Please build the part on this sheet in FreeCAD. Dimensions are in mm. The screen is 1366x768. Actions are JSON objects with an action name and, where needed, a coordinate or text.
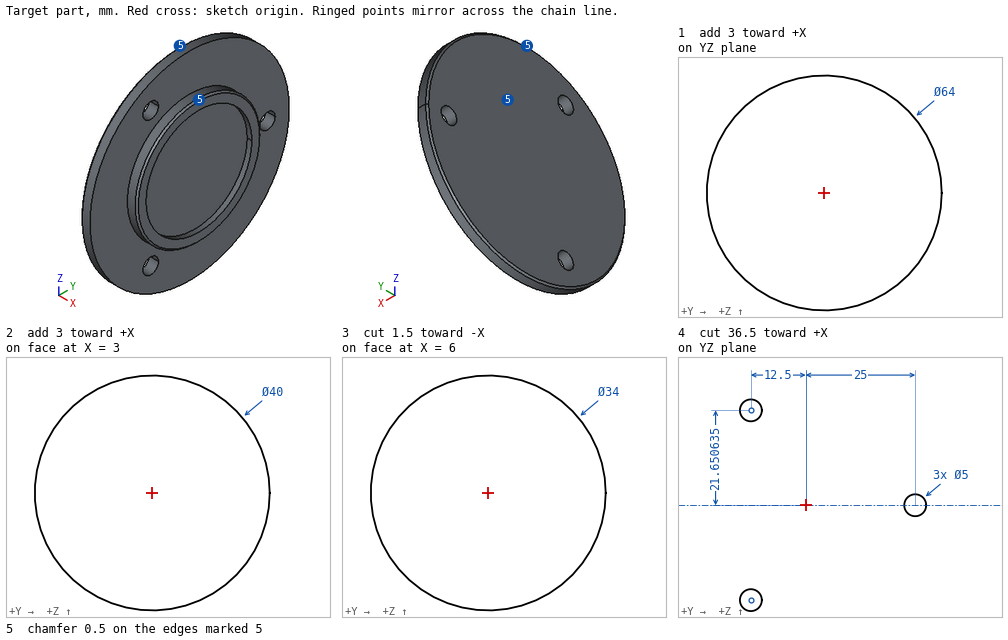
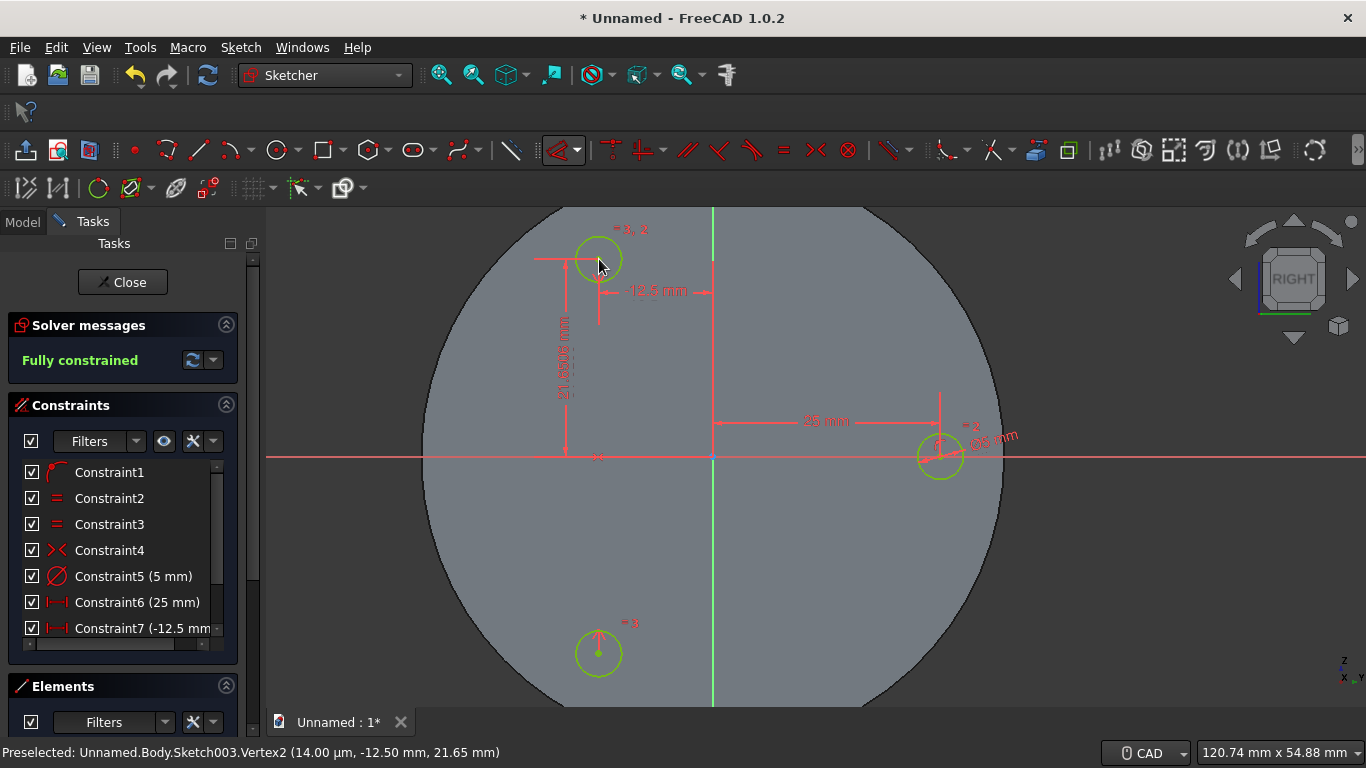
{"action": "left_click", "coordinate": [123, 282]}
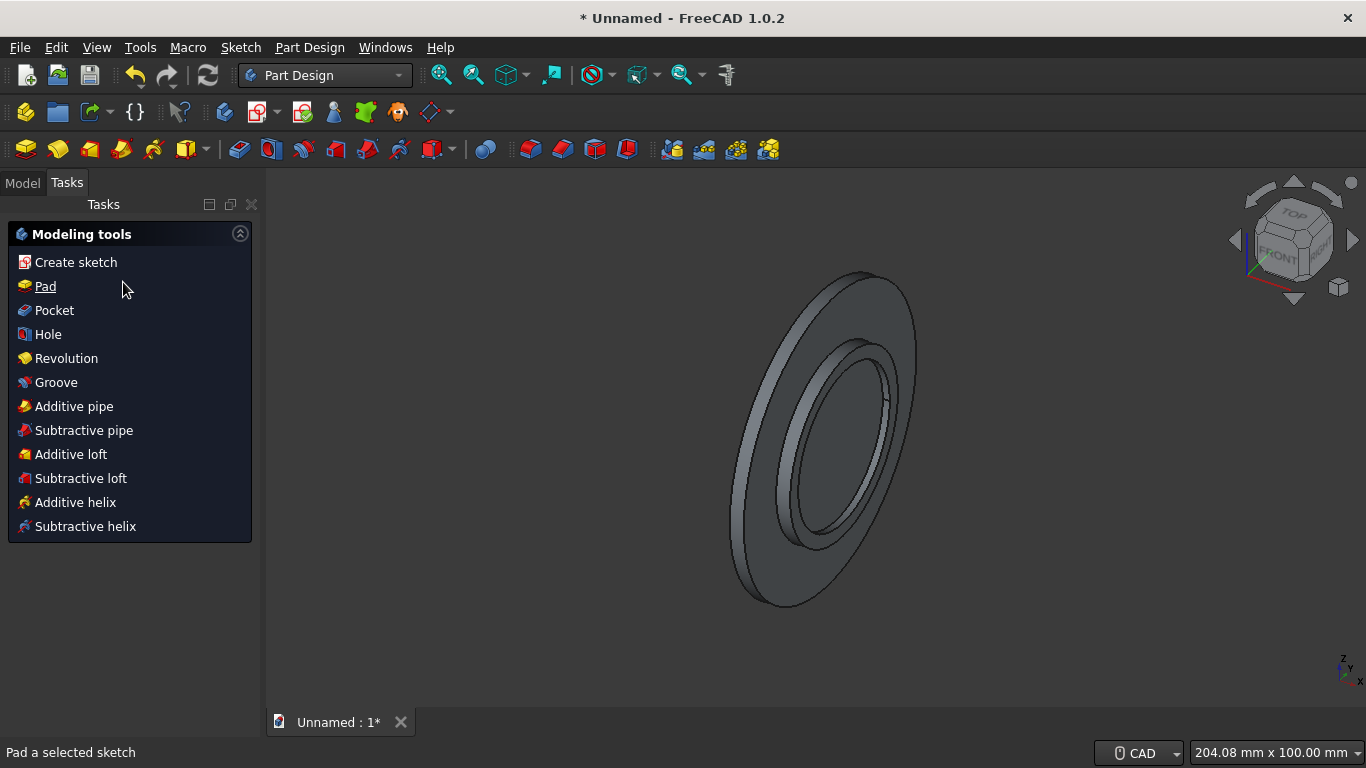
{"action": "left_click", "coordinate": [240, 150]}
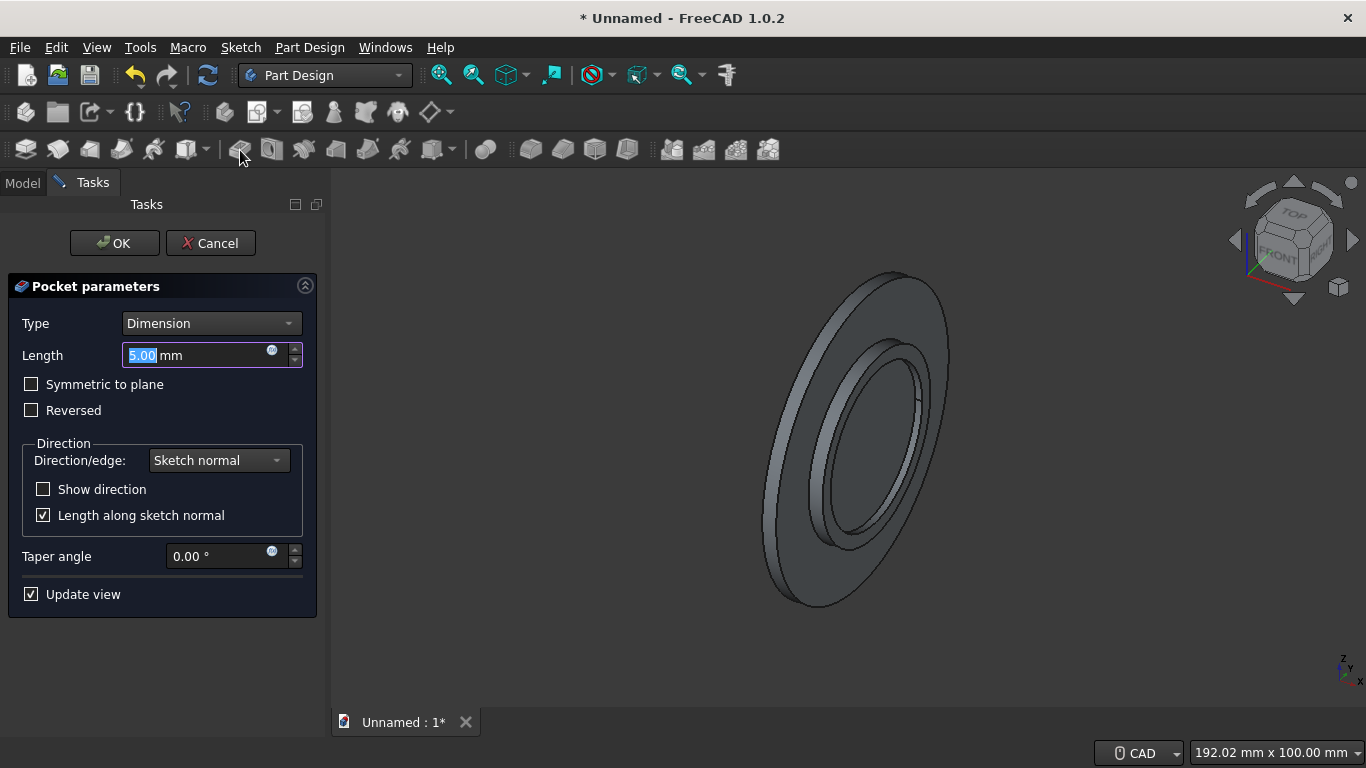
{"action": "type", "text": "36.5"}
{"action": "key", "text": "Tab"}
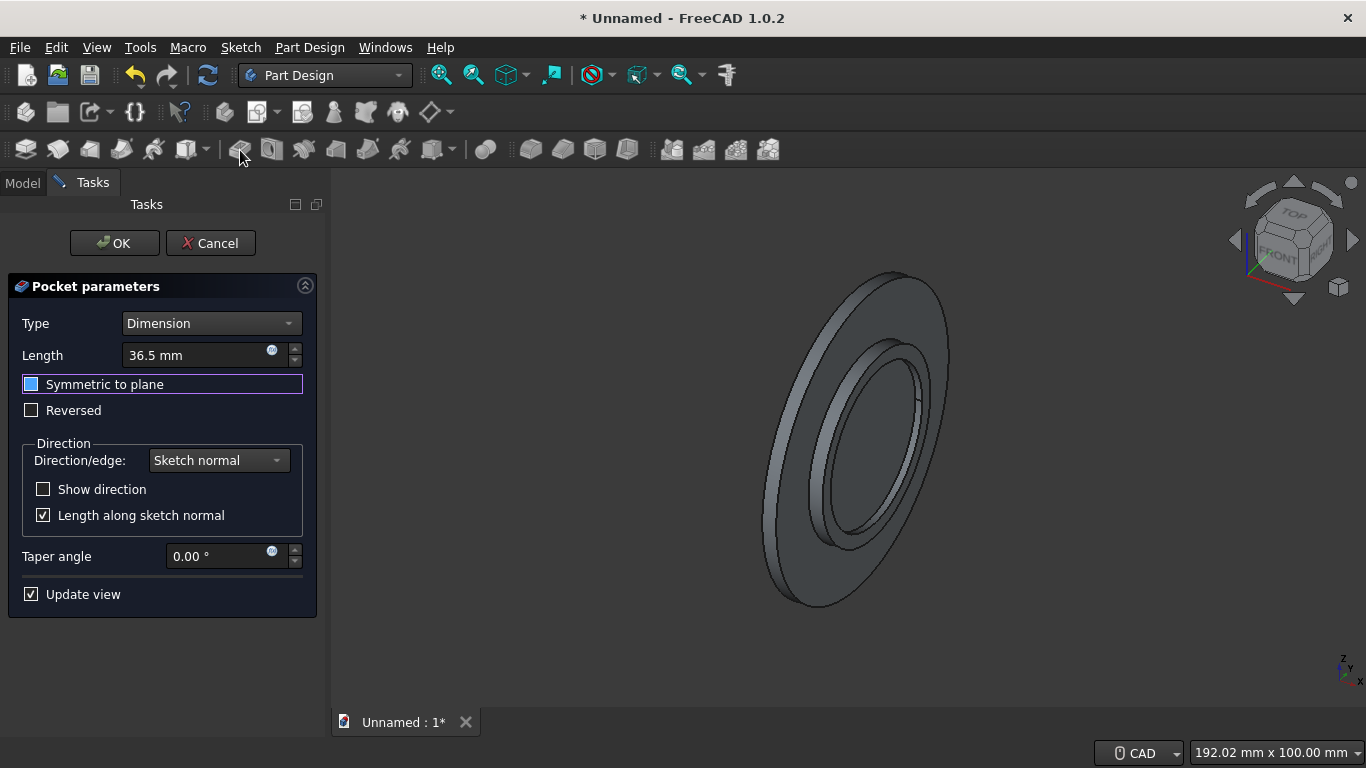
{"action": "left_click", "coordinate": [30, 410]}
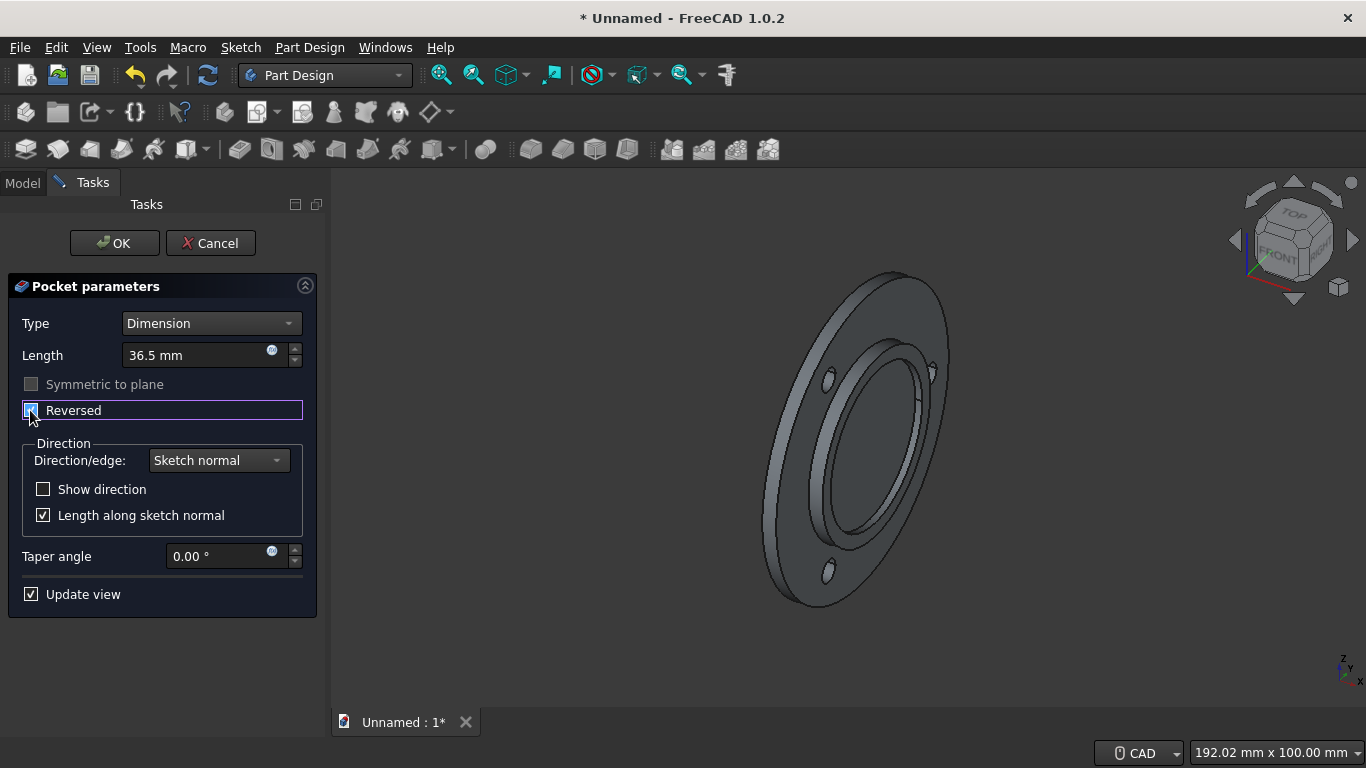
{"action": "left_click", "coordinate": [115, 243]}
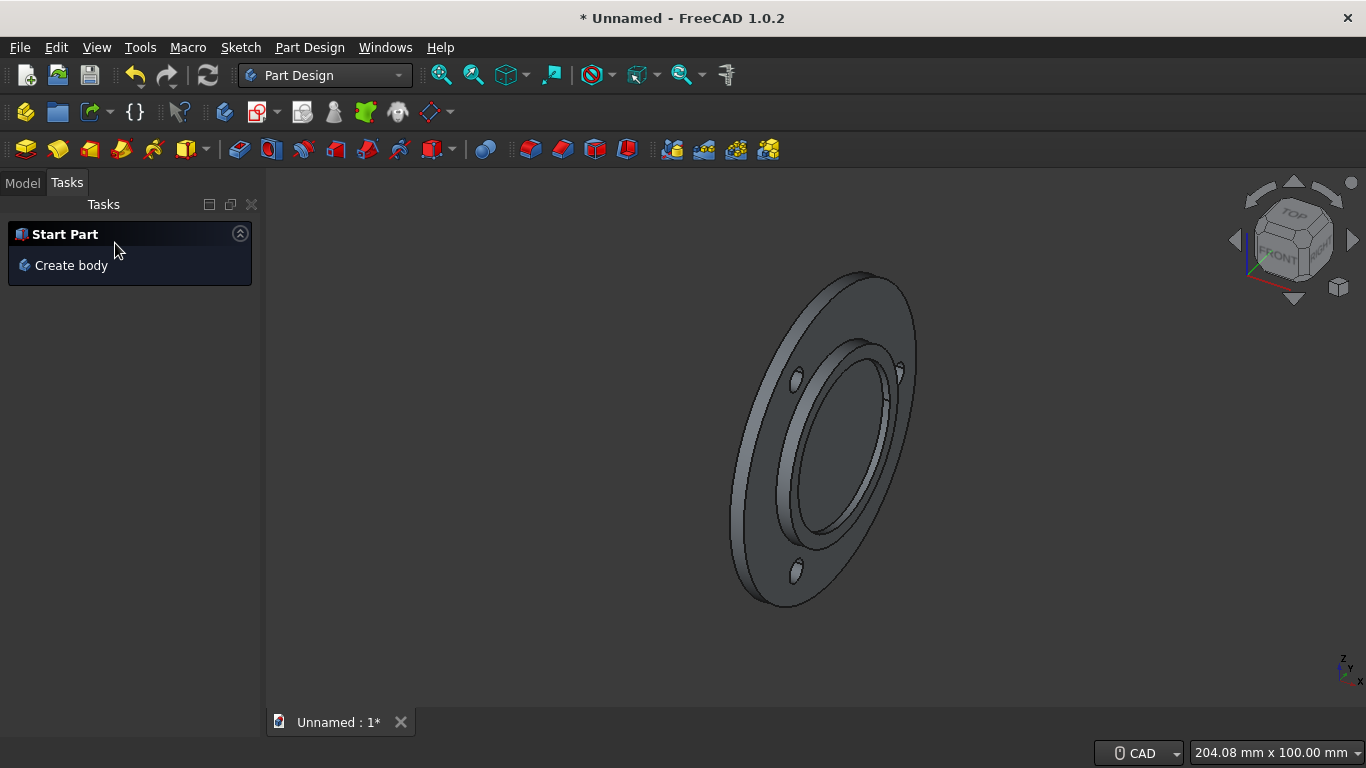
{"action": "left_click", "coordinate": [790, 499]}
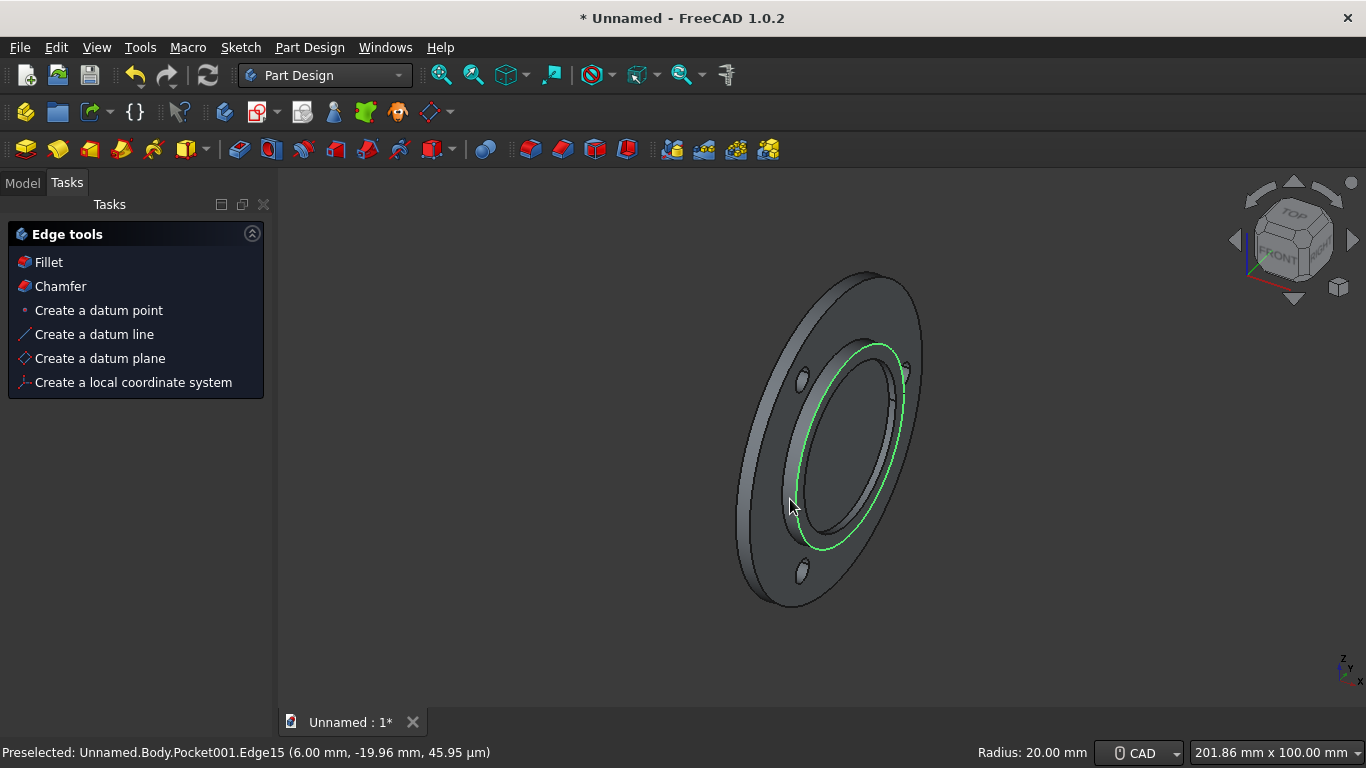
{"action": "key", "text": "0"}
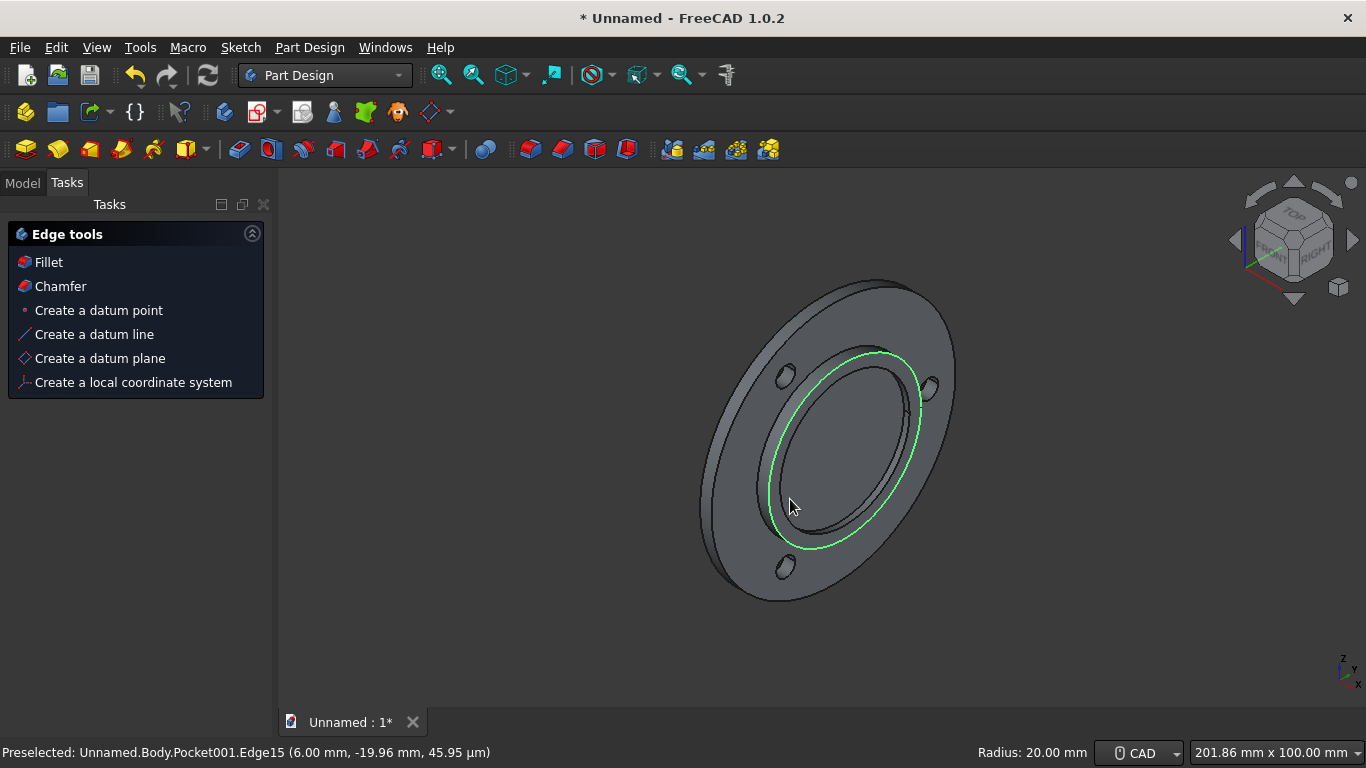
{"action": "key", "text": "2"}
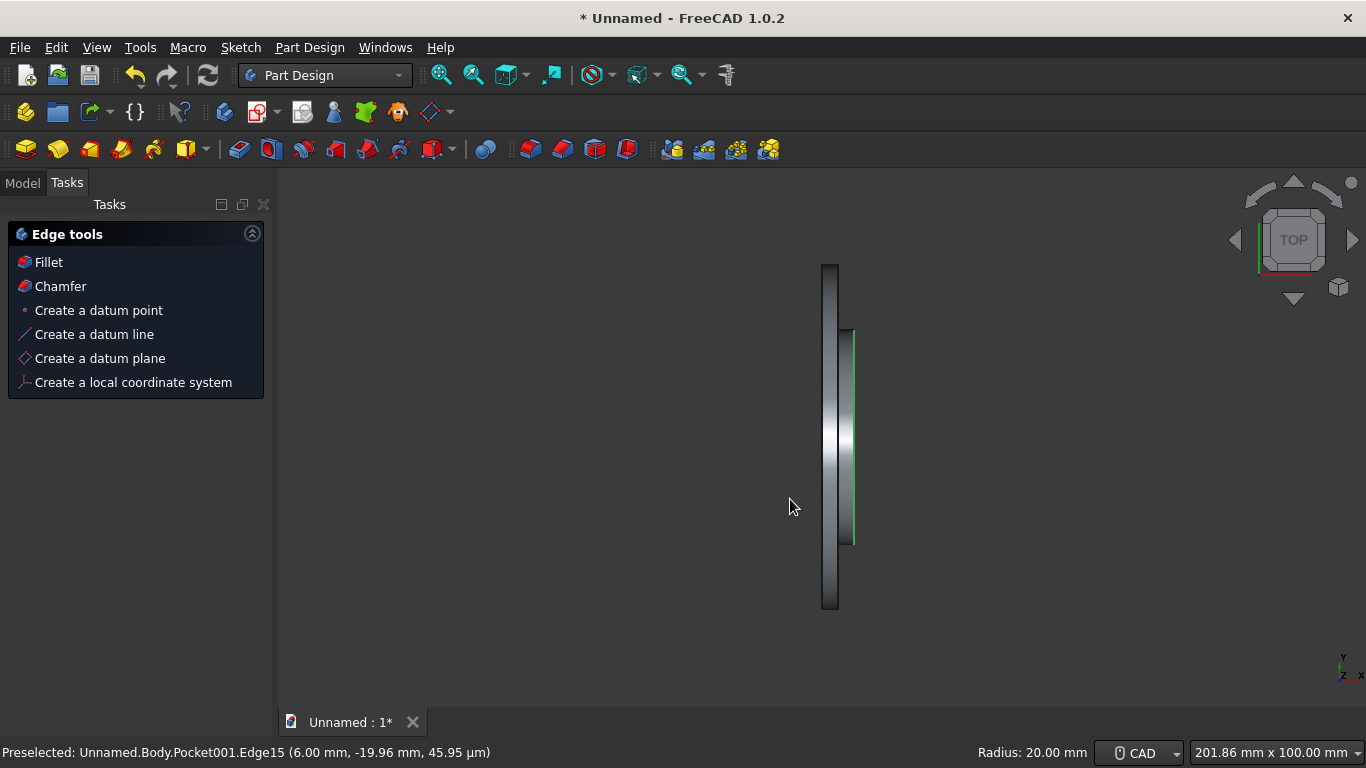
{"action": "left_click", "coordinate": [822, 576], "text": "ctrl"}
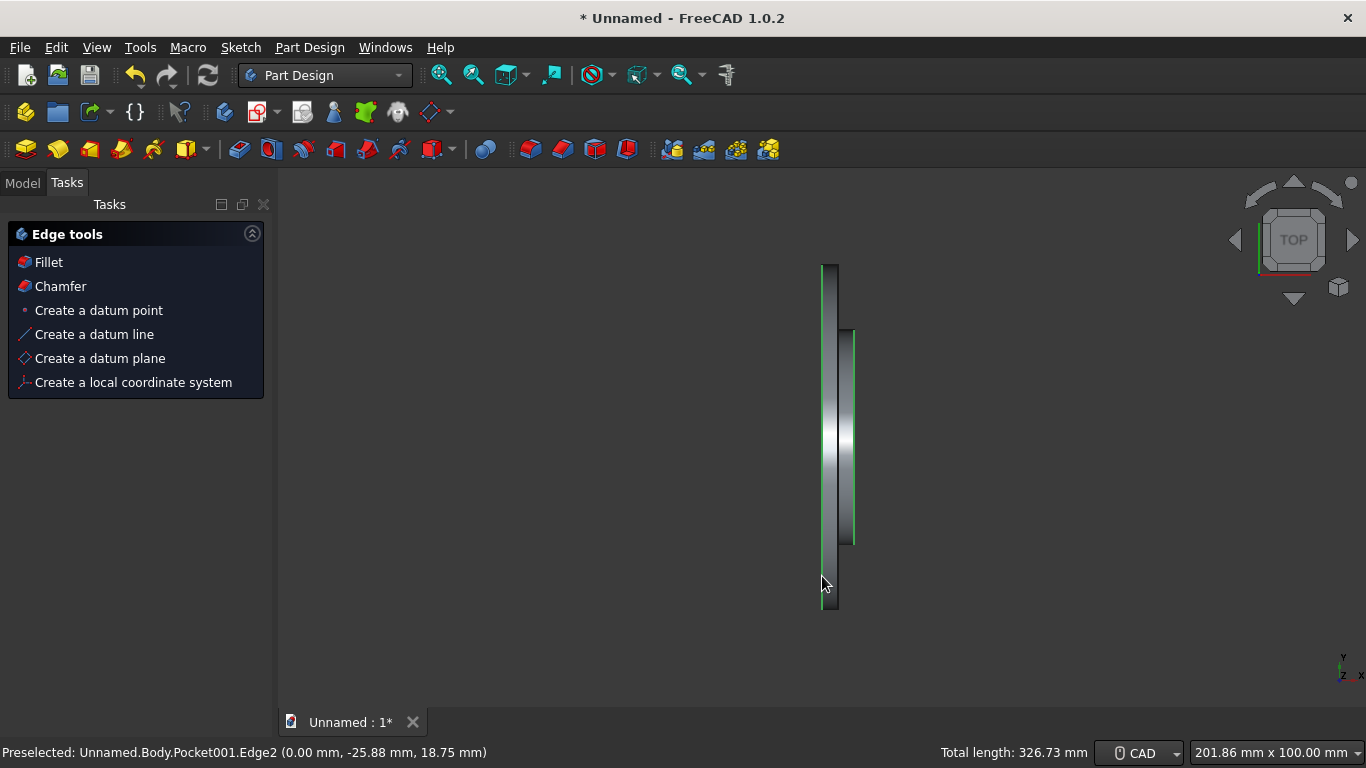
{"action": "left_click", "coordinate": [564, 150]}